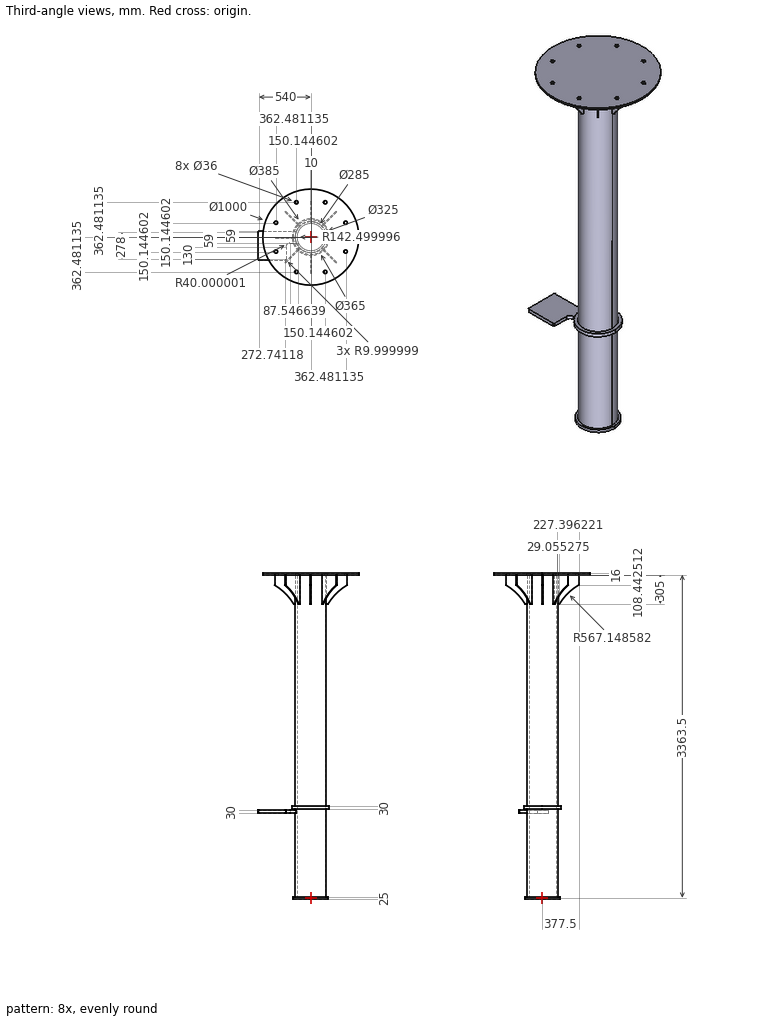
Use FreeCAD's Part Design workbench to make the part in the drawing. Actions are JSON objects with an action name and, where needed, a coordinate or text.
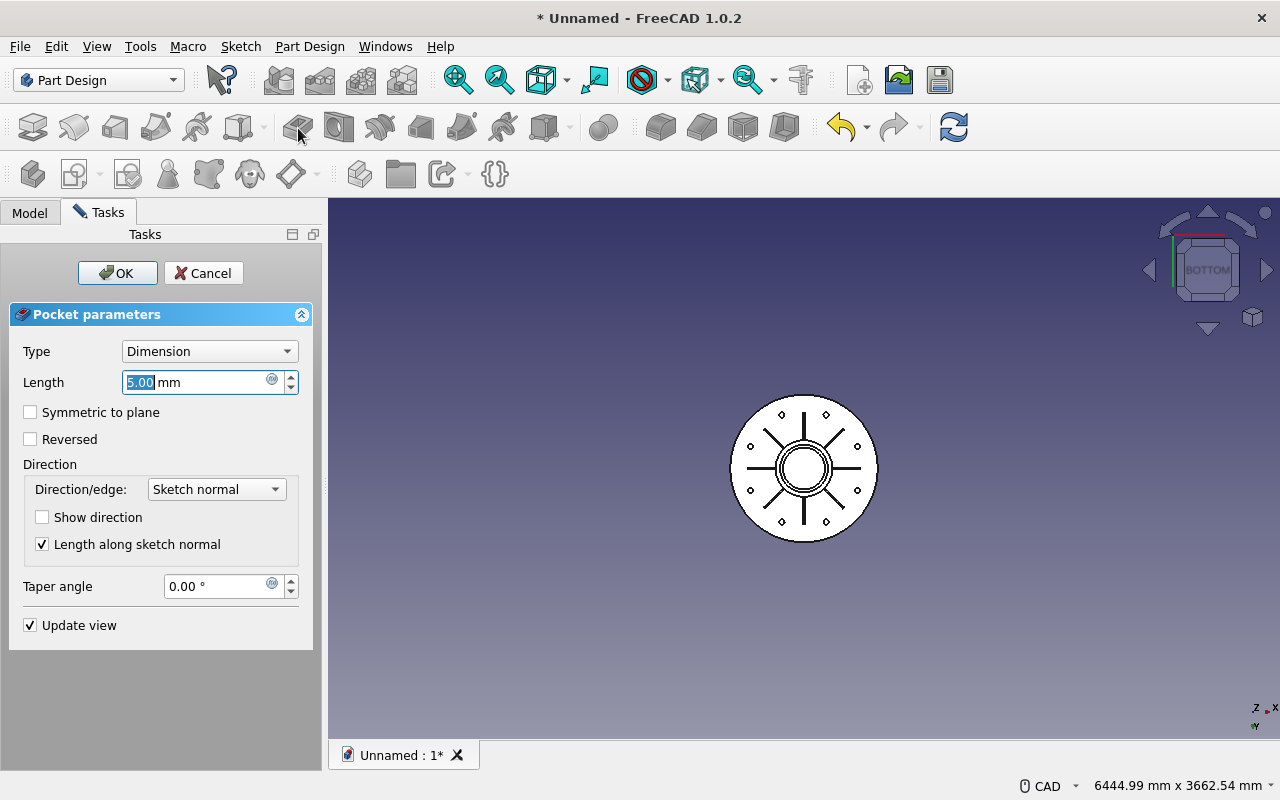
{"action": "left_click", "coordinate": [210, 352]}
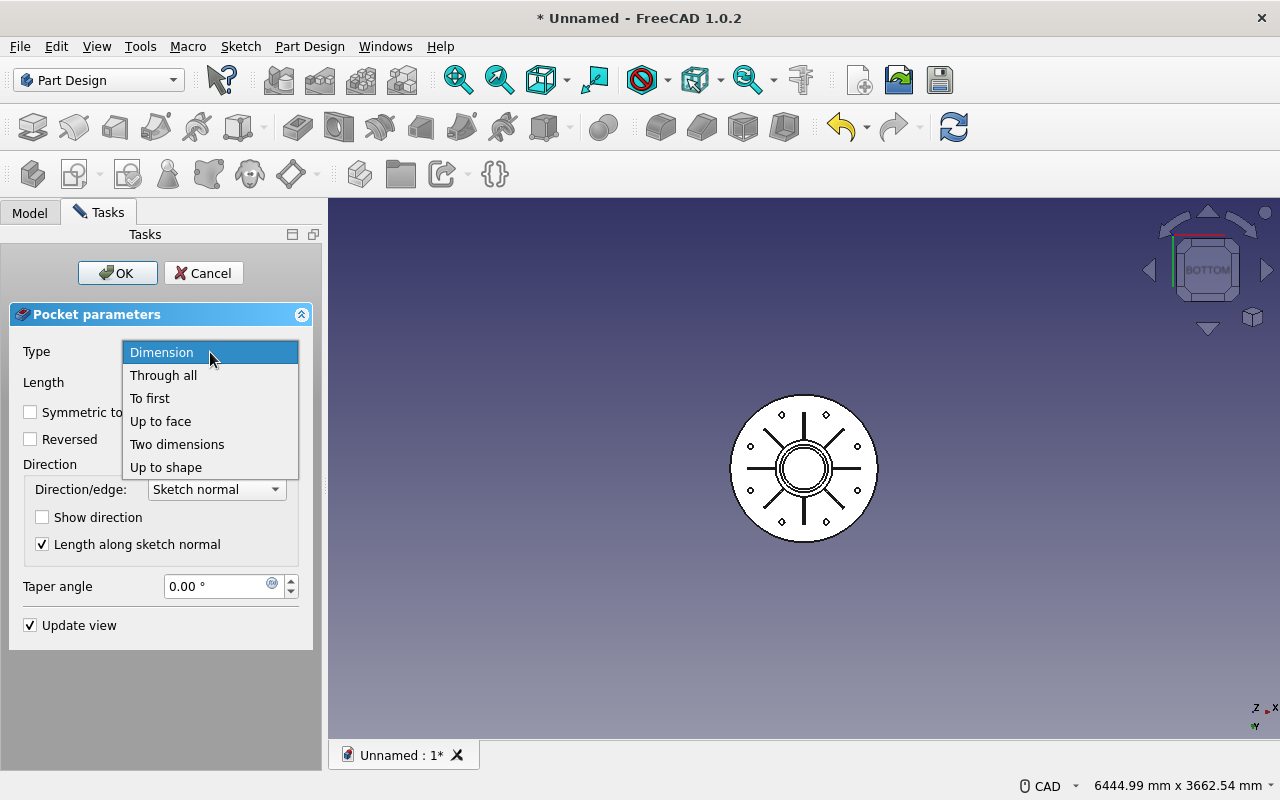
{"action": "left_click", "coordinate": [208, 376]}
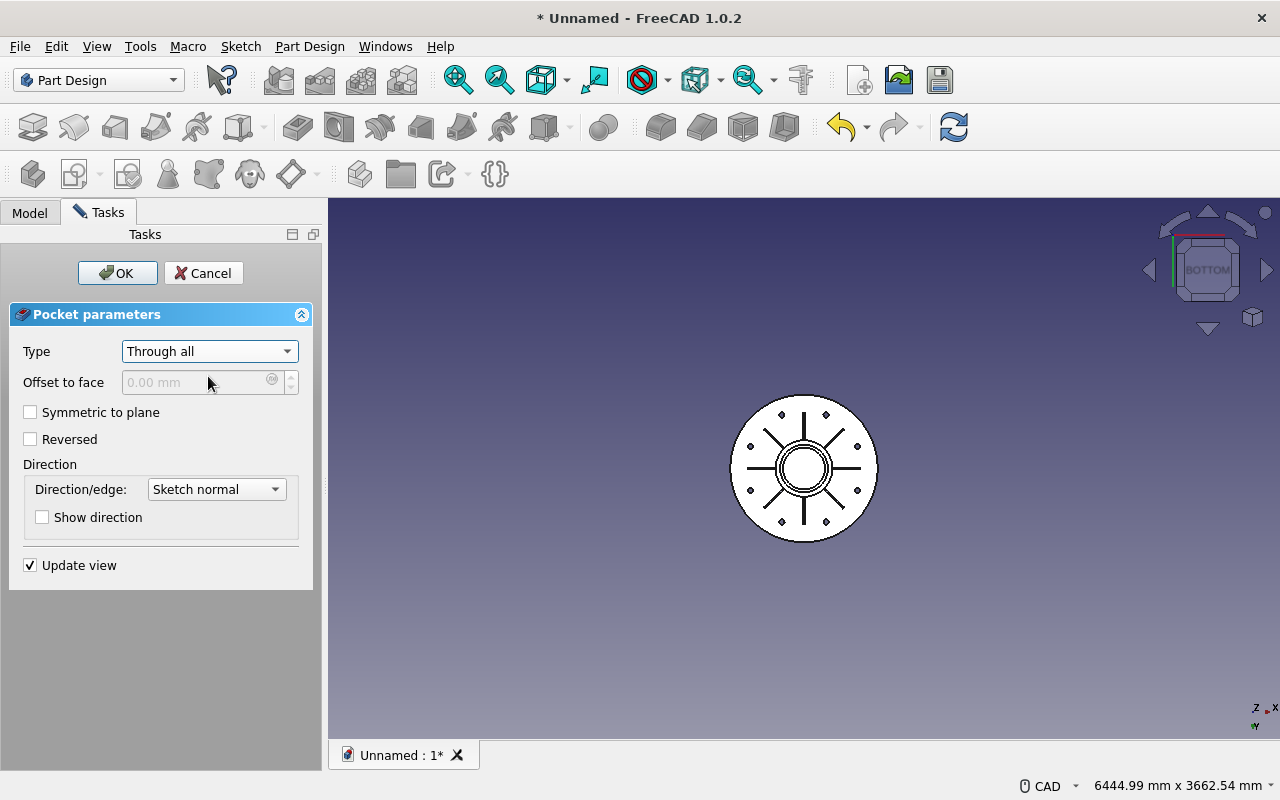
{"action": "left_click", "coordinate": [118, 273]}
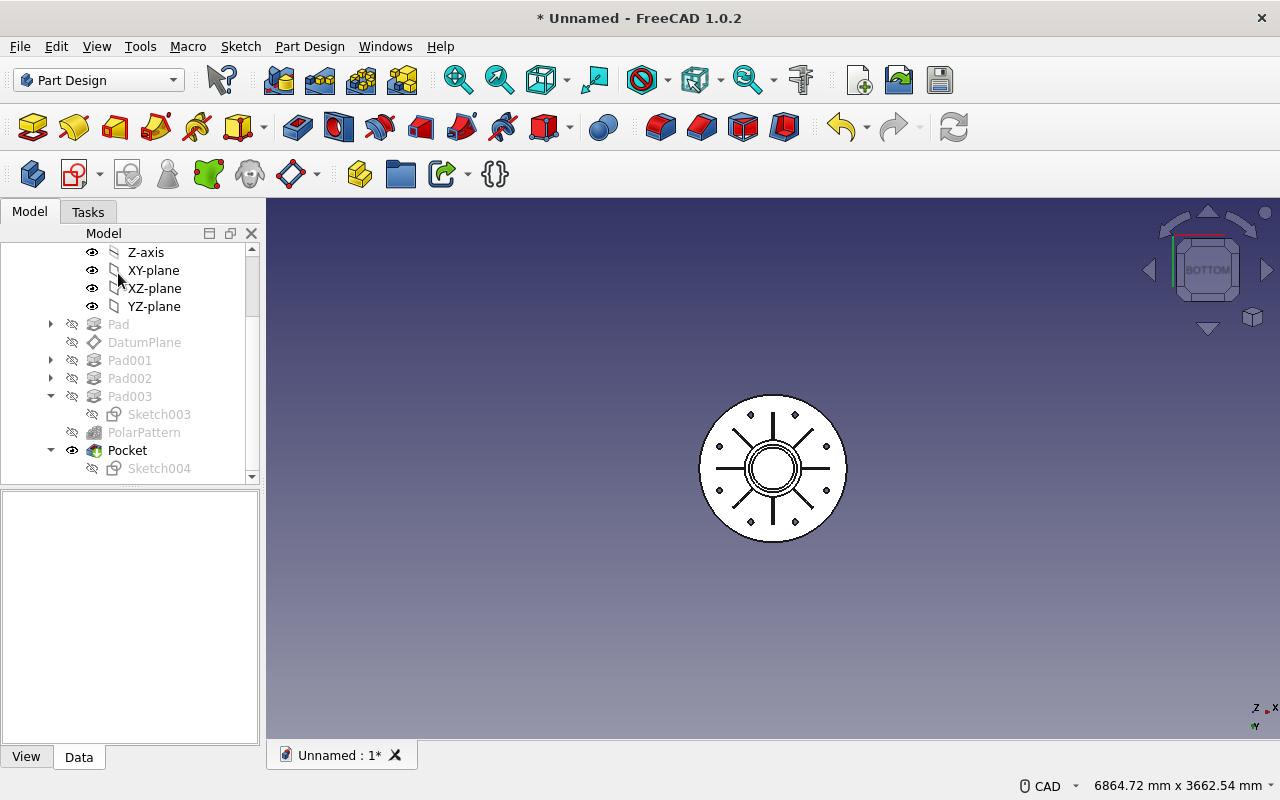
{"action": "key", "text": "v f"}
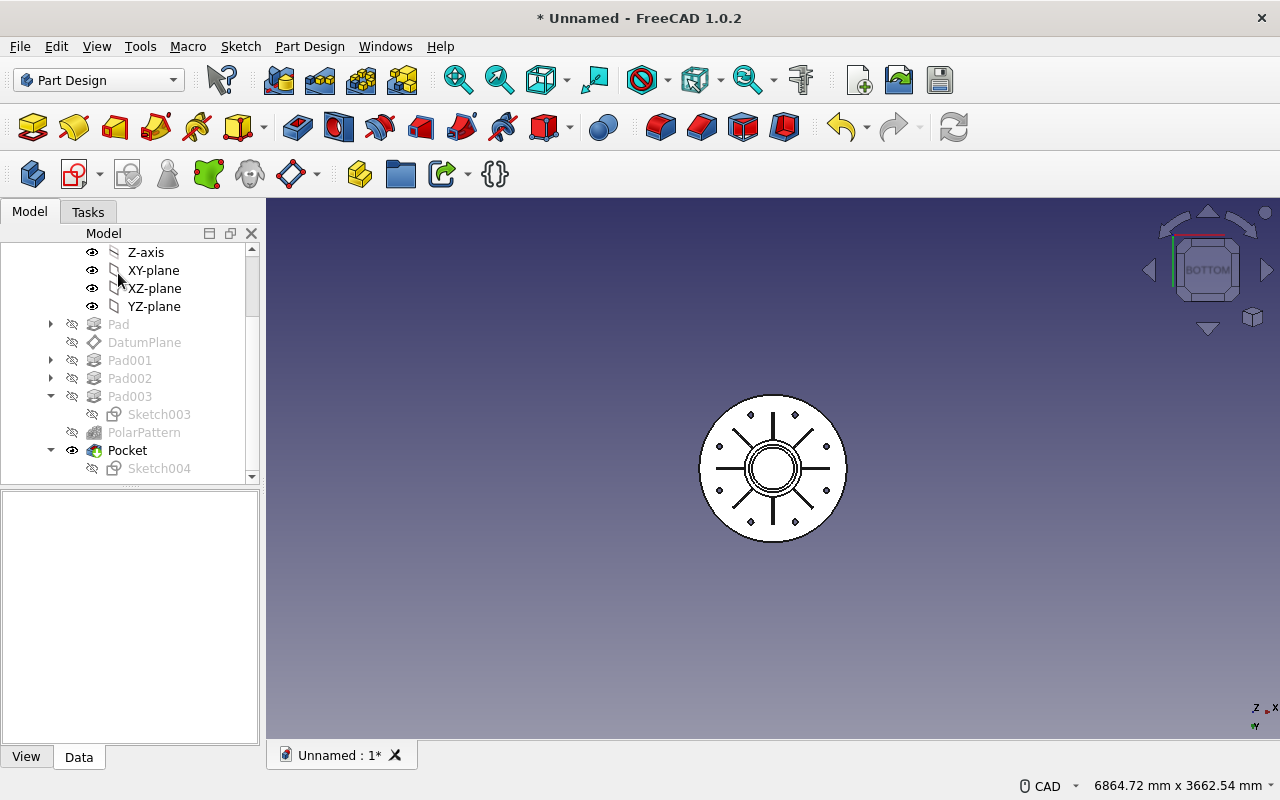
{"action": "scroll", "coordinate": [794, 474], "scroll_direction": "up", "scroll_amount": 15}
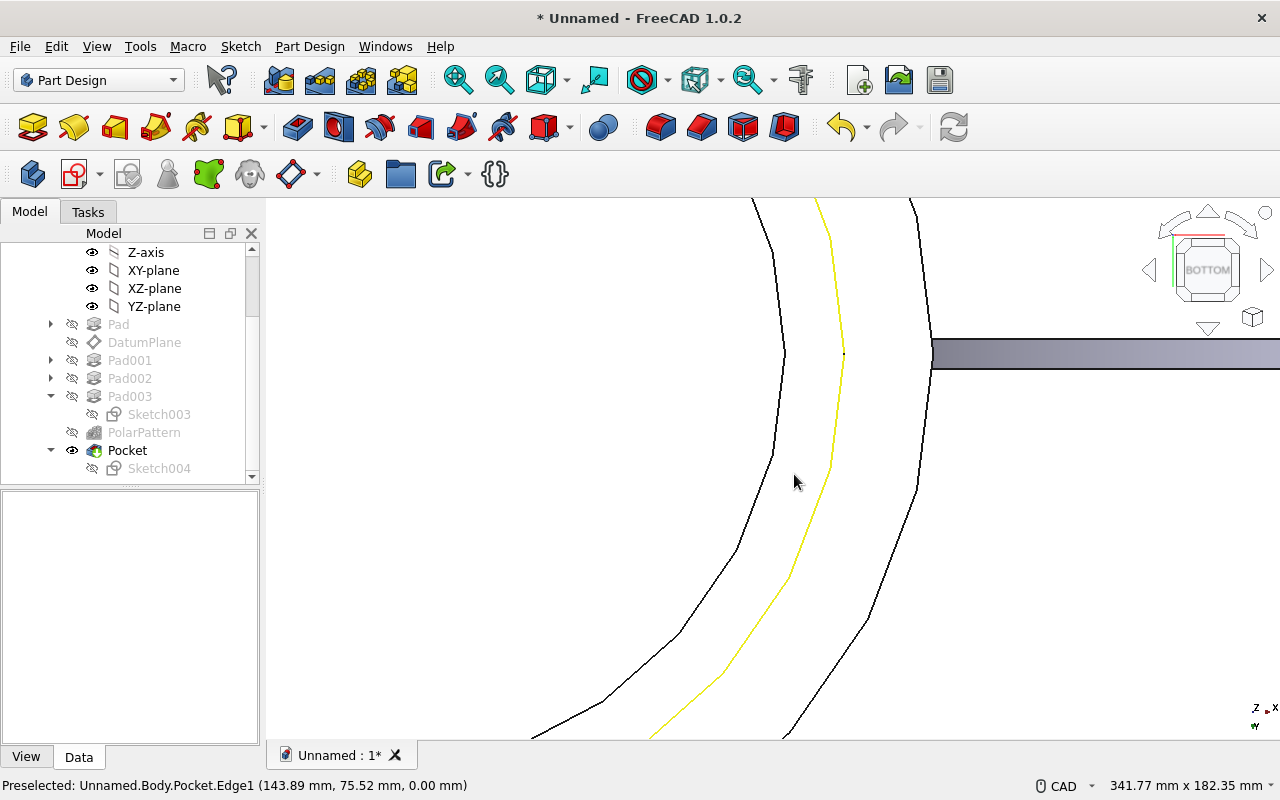
{"action": "left_click", "coordinate": [775, 491]}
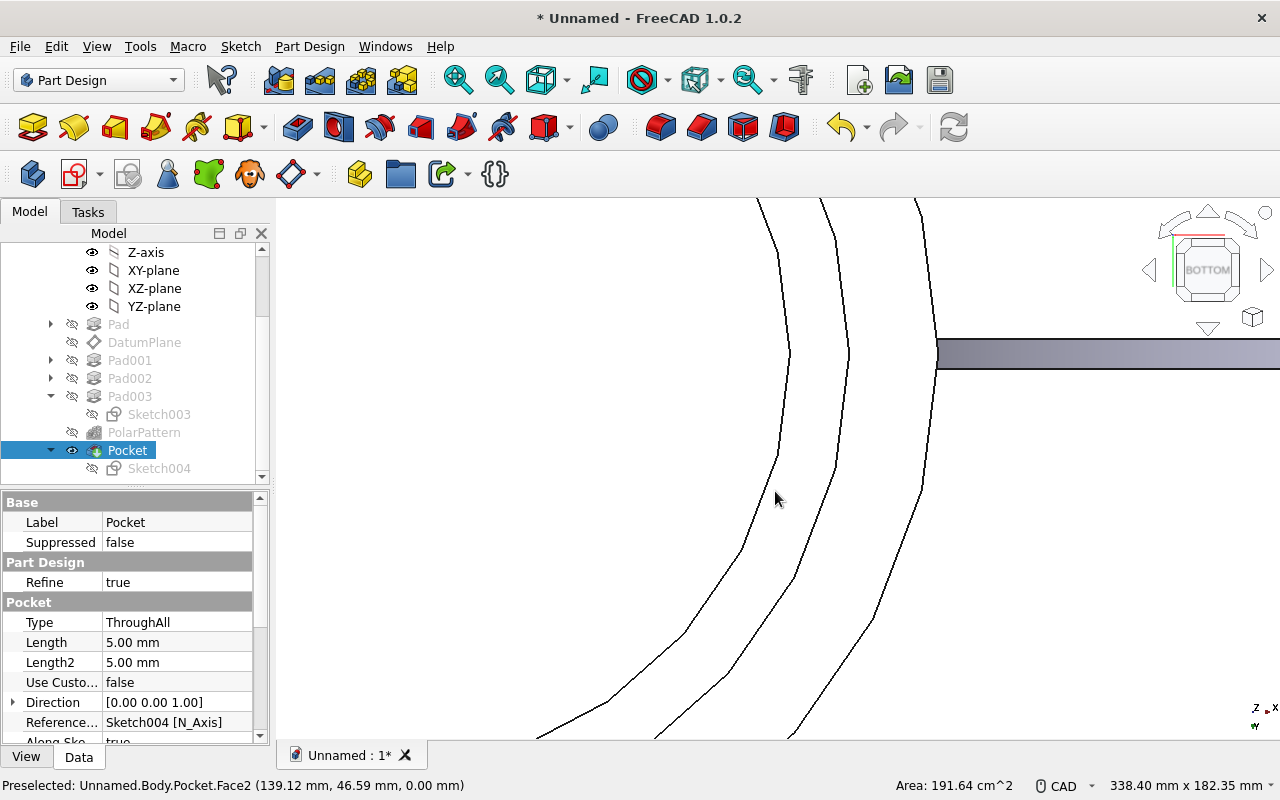
{"action": "left_click", "coordinate": [74, 174]}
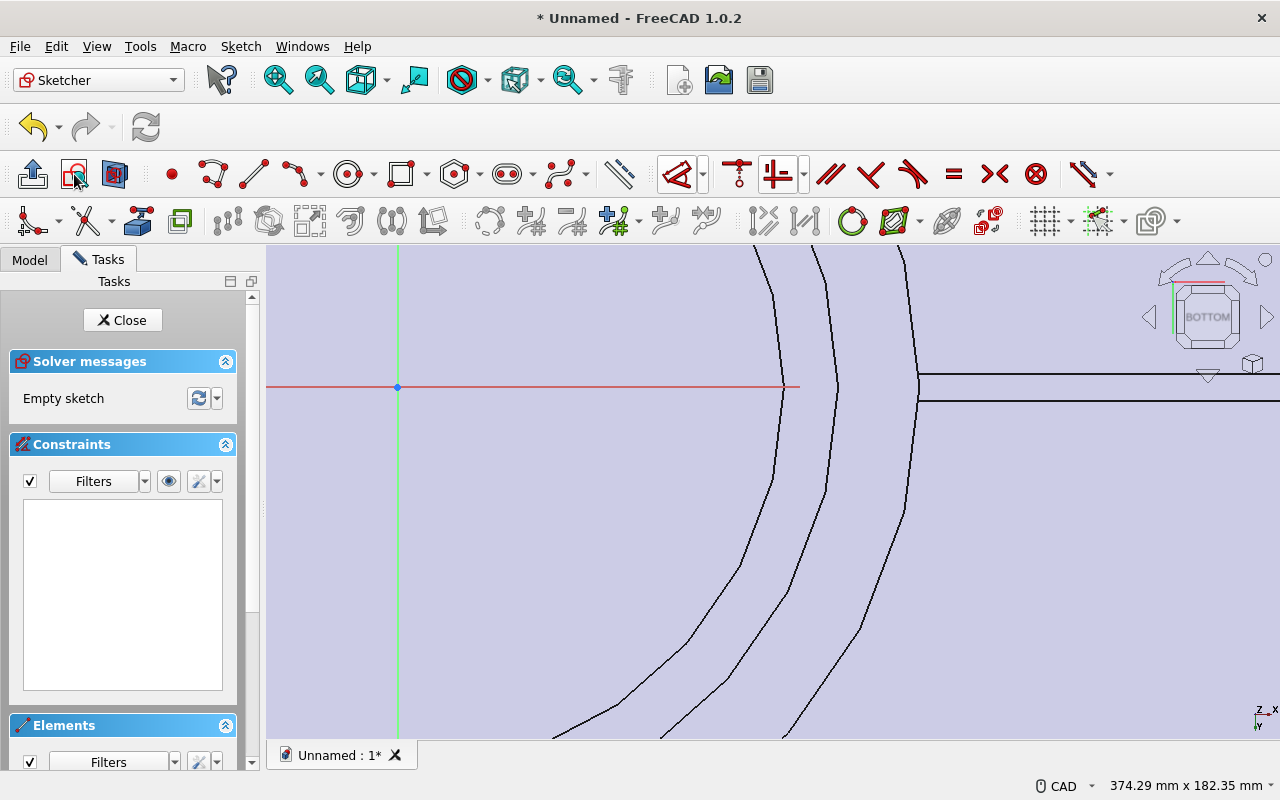
{"action": "scroll", "coordinate": [837, 537], "scroll_direction": "down", "scroll_amount": 6}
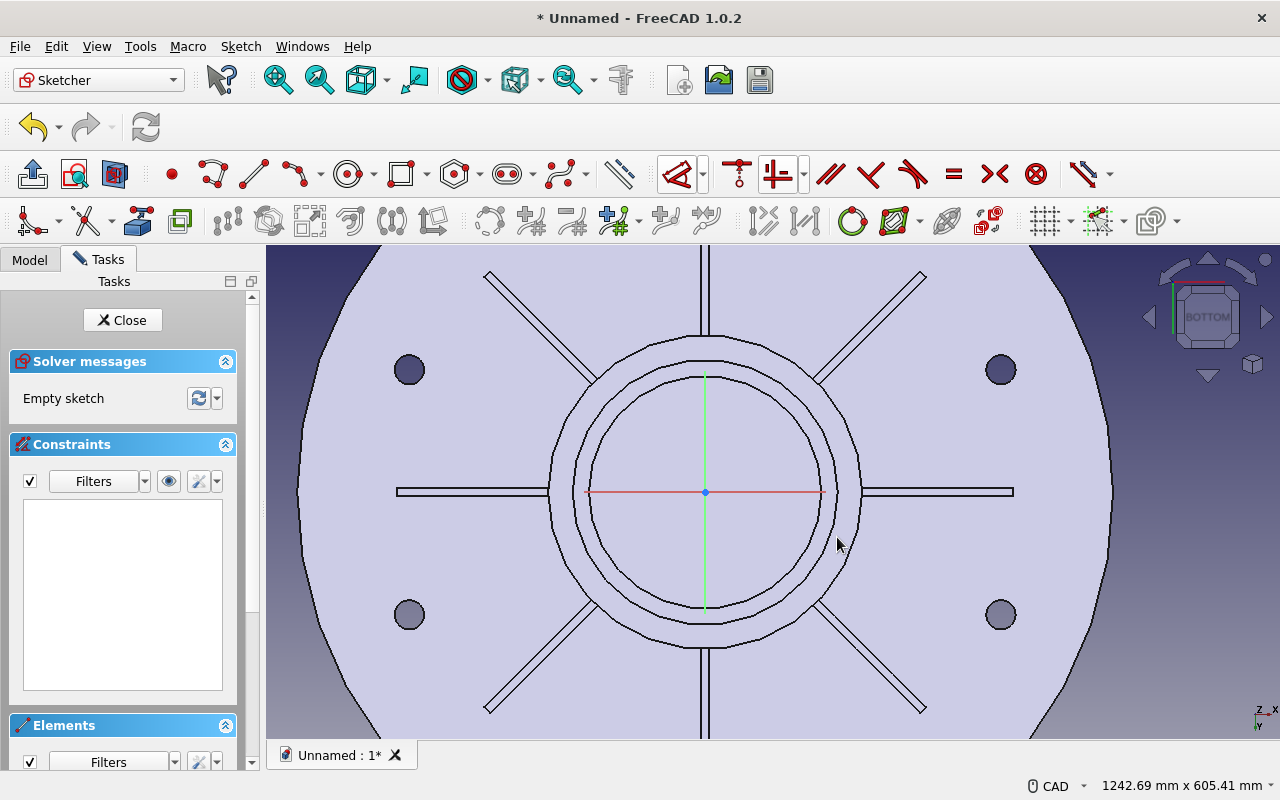
{"action": "left_click", "coordinate": [348, 174]}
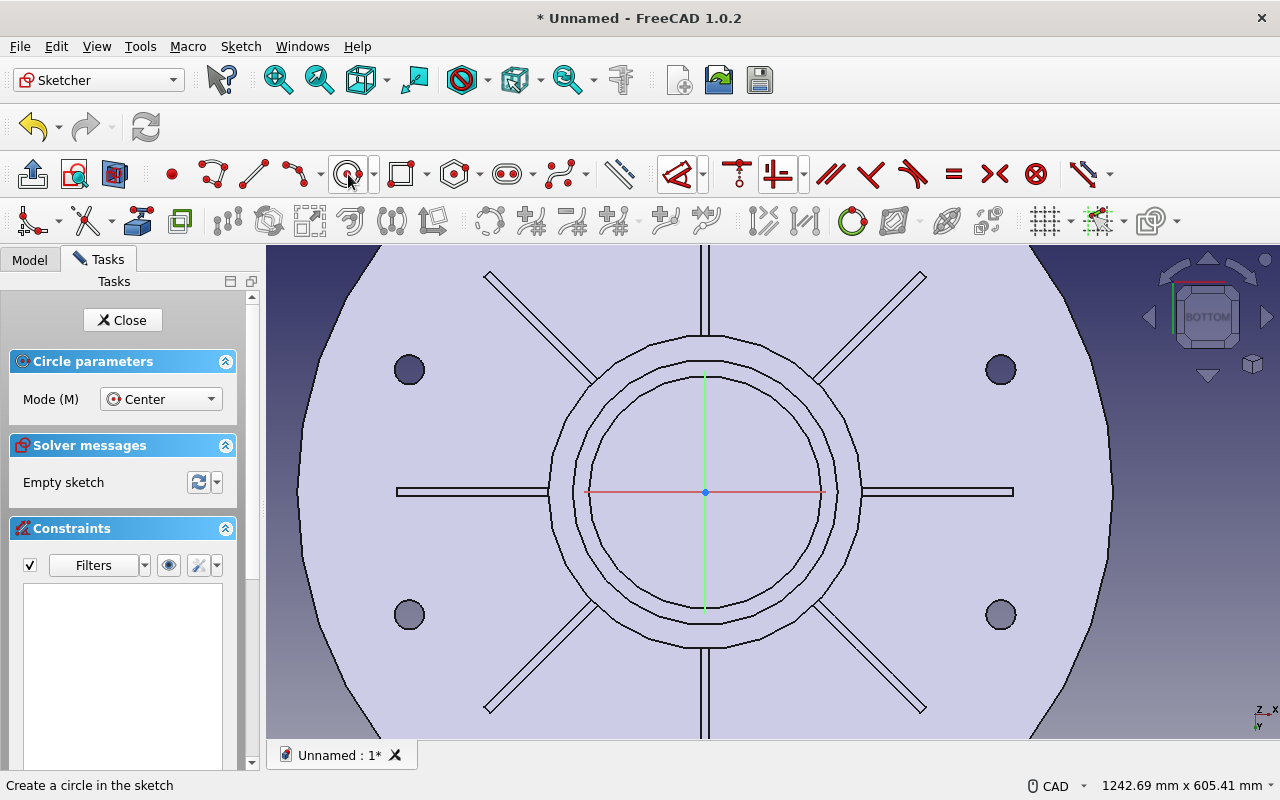
{"action": "left_click", "coordinate": [705, 492]}
{"action": "left_click", "coordinate": [810, 387]}
{"action": "key", "text": "Escape"}